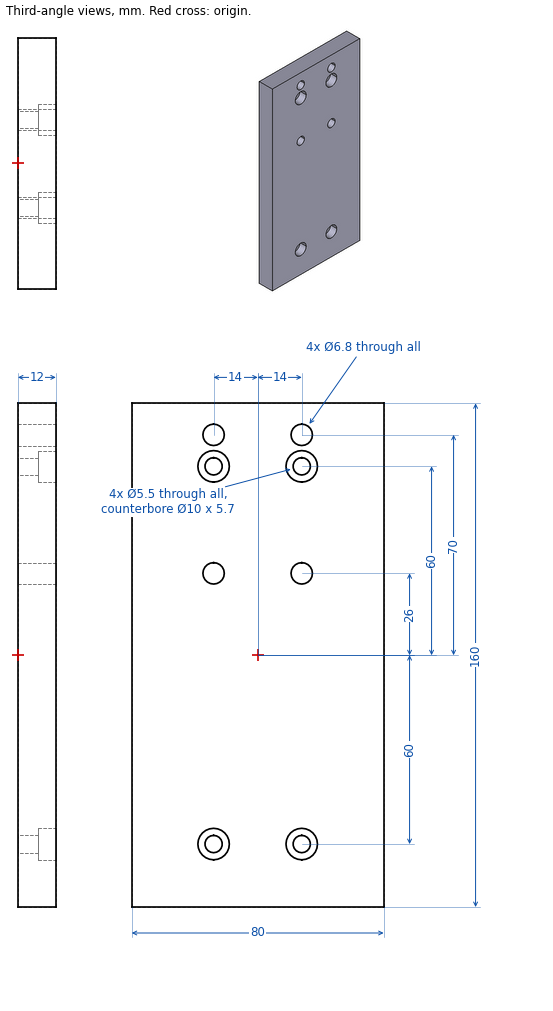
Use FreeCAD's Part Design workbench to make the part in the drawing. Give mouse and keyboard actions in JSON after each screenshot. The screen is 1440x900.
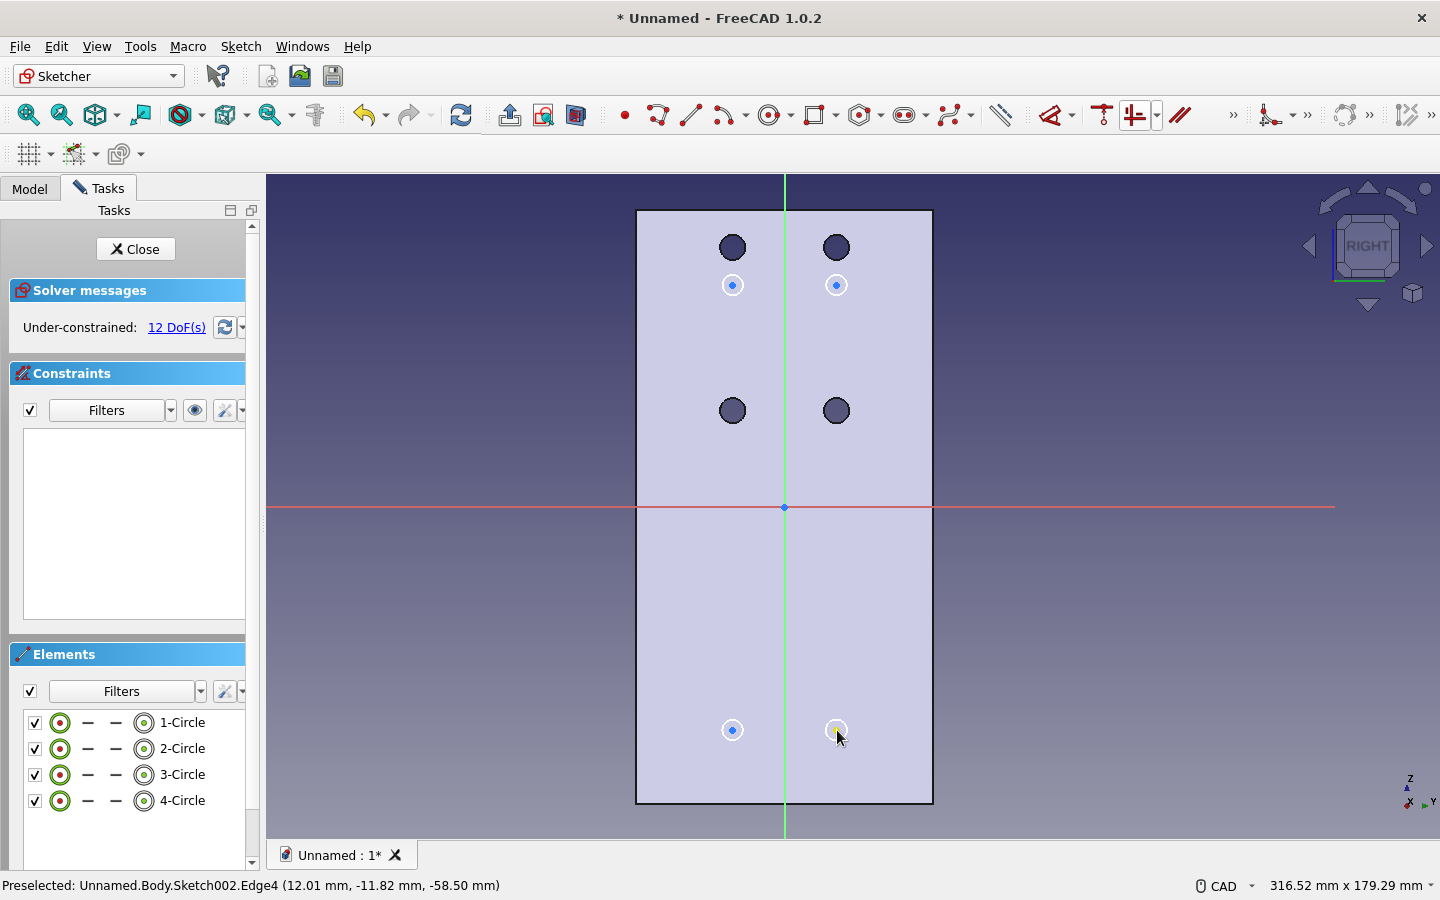
{"action": "scroll", "coordinate": [844, 278], "scroll_direction": "up", "scroll_amount": 2}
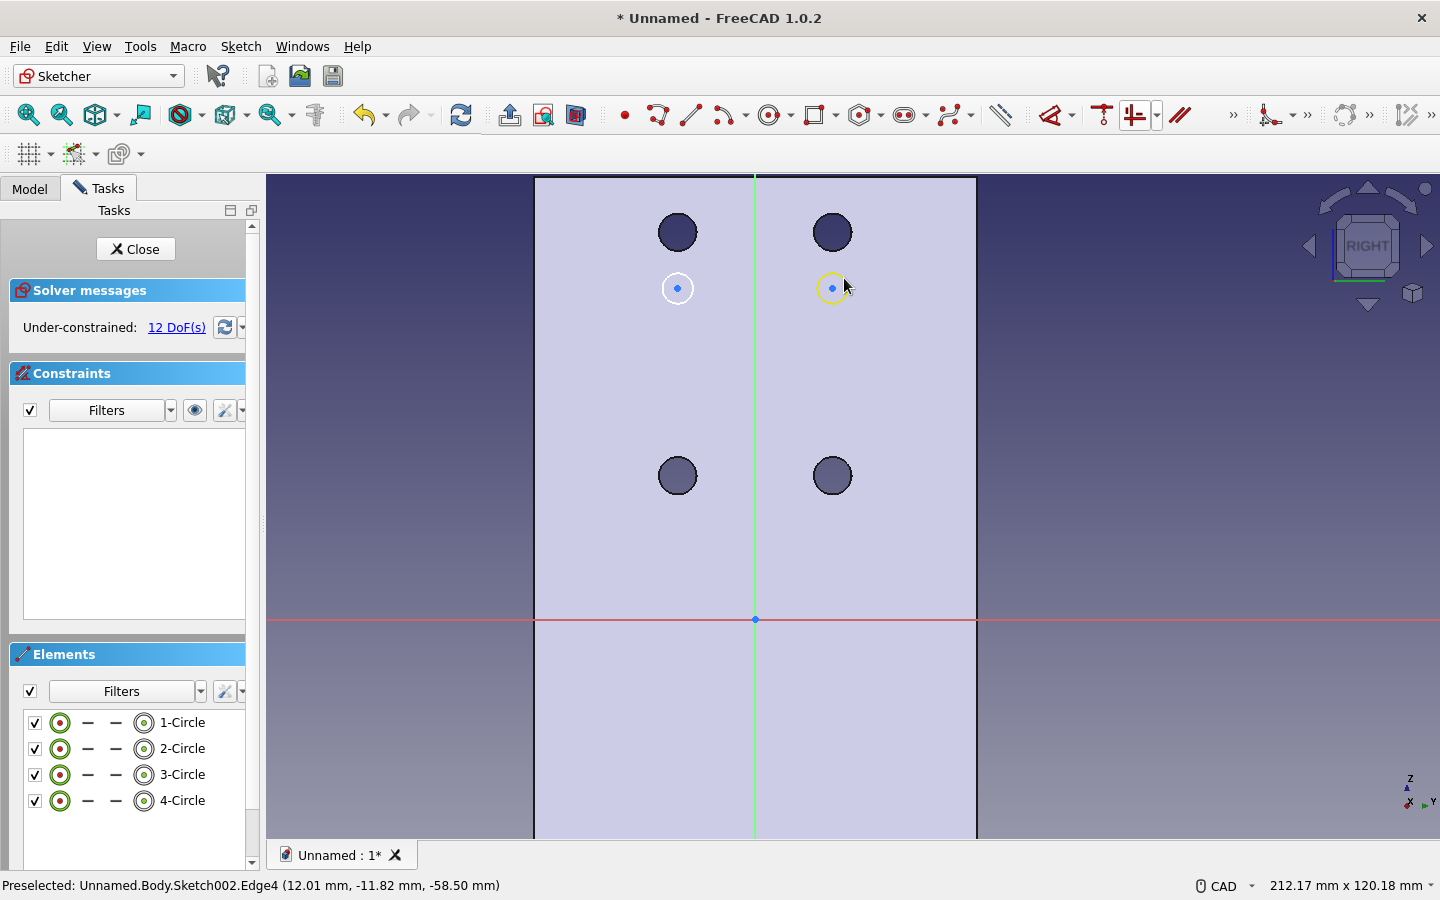
{"action": "left_click", "coordinate": [843, 278]}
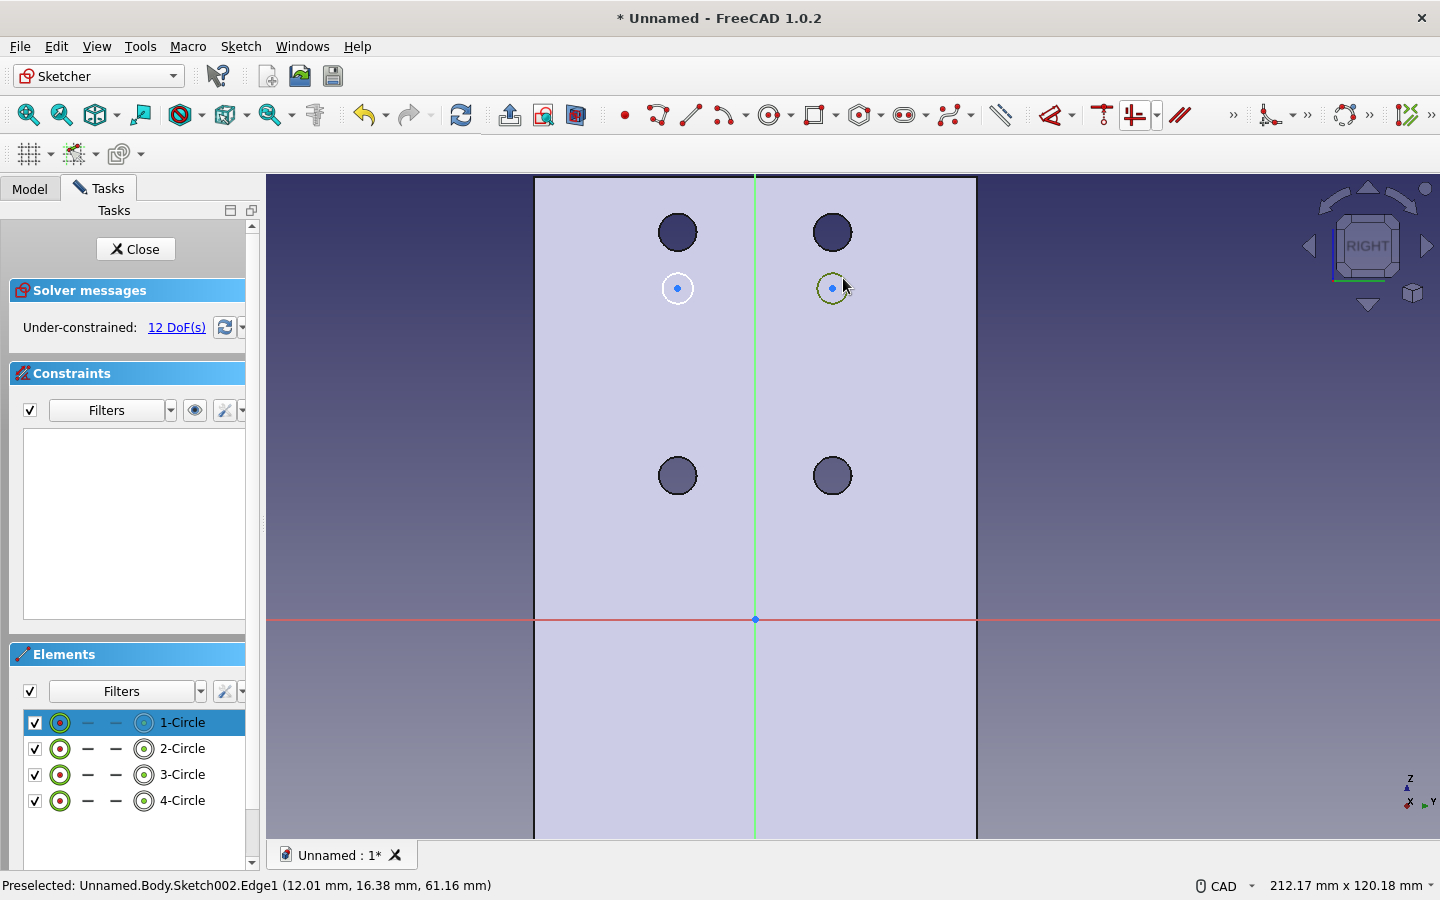
{"action": "left_click", "coordinate": [688, 278]}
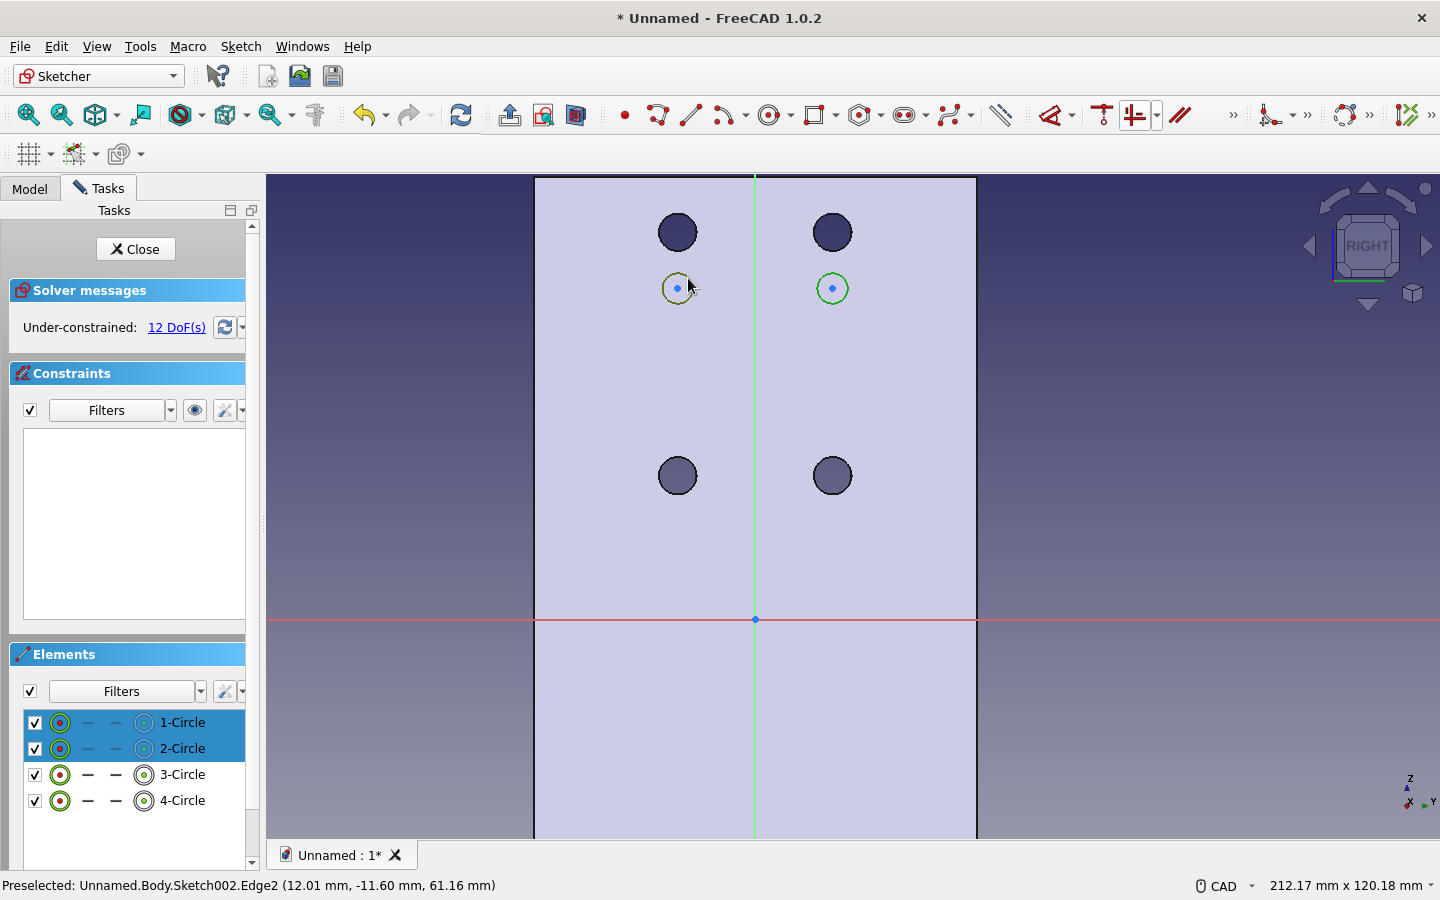
{"action": "scroll", "coordinate": [844, 276], "scroll_direction": "down", "scroll_amount": 2}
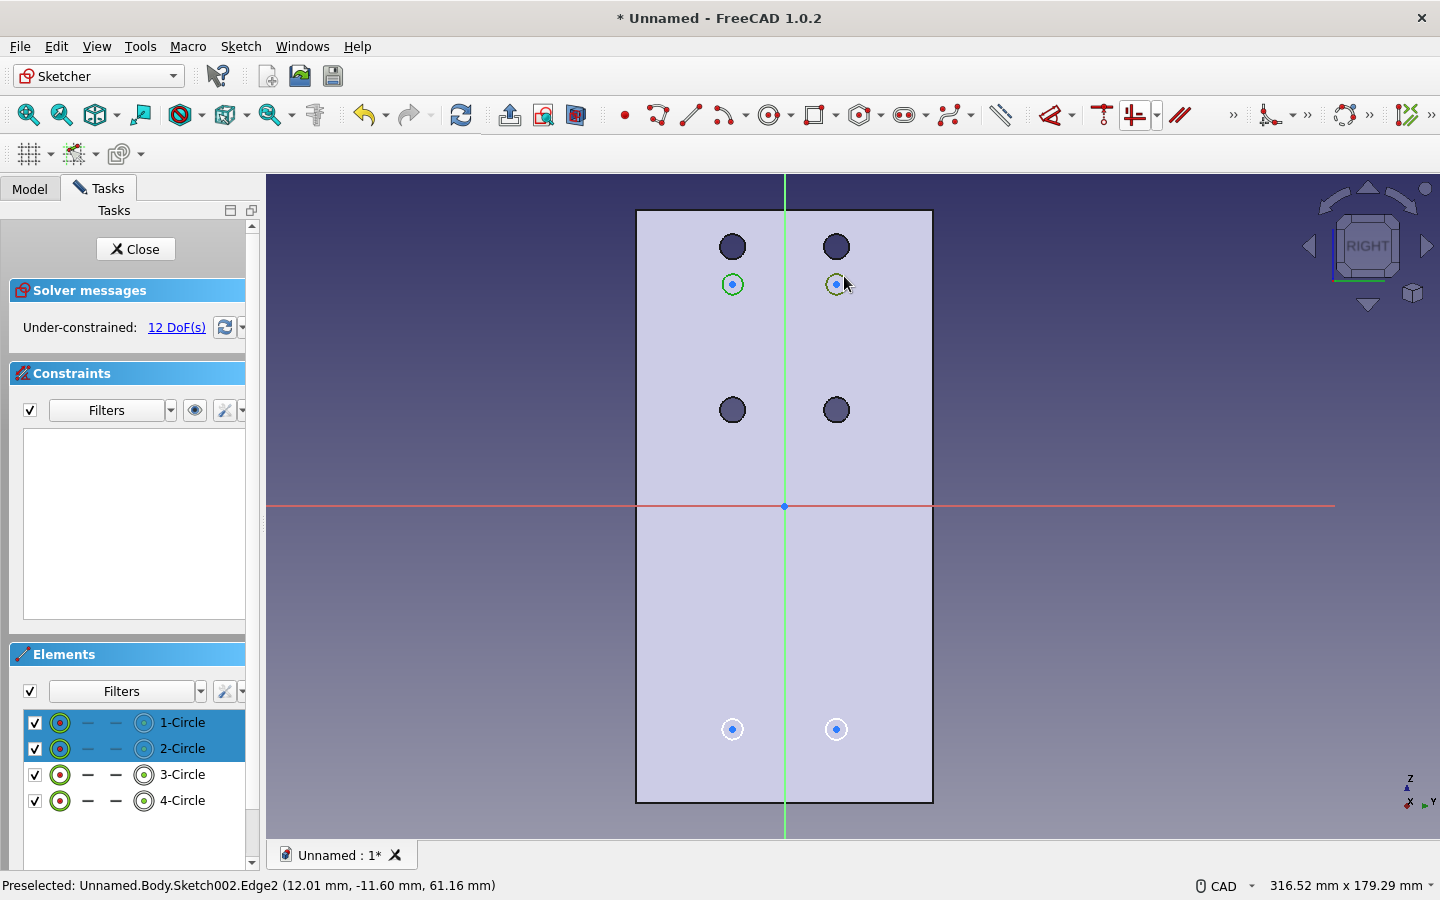
{"action": "scroll", "coordinate": [844, 722], "scroll_direction": "up", "scroll_amount": 2}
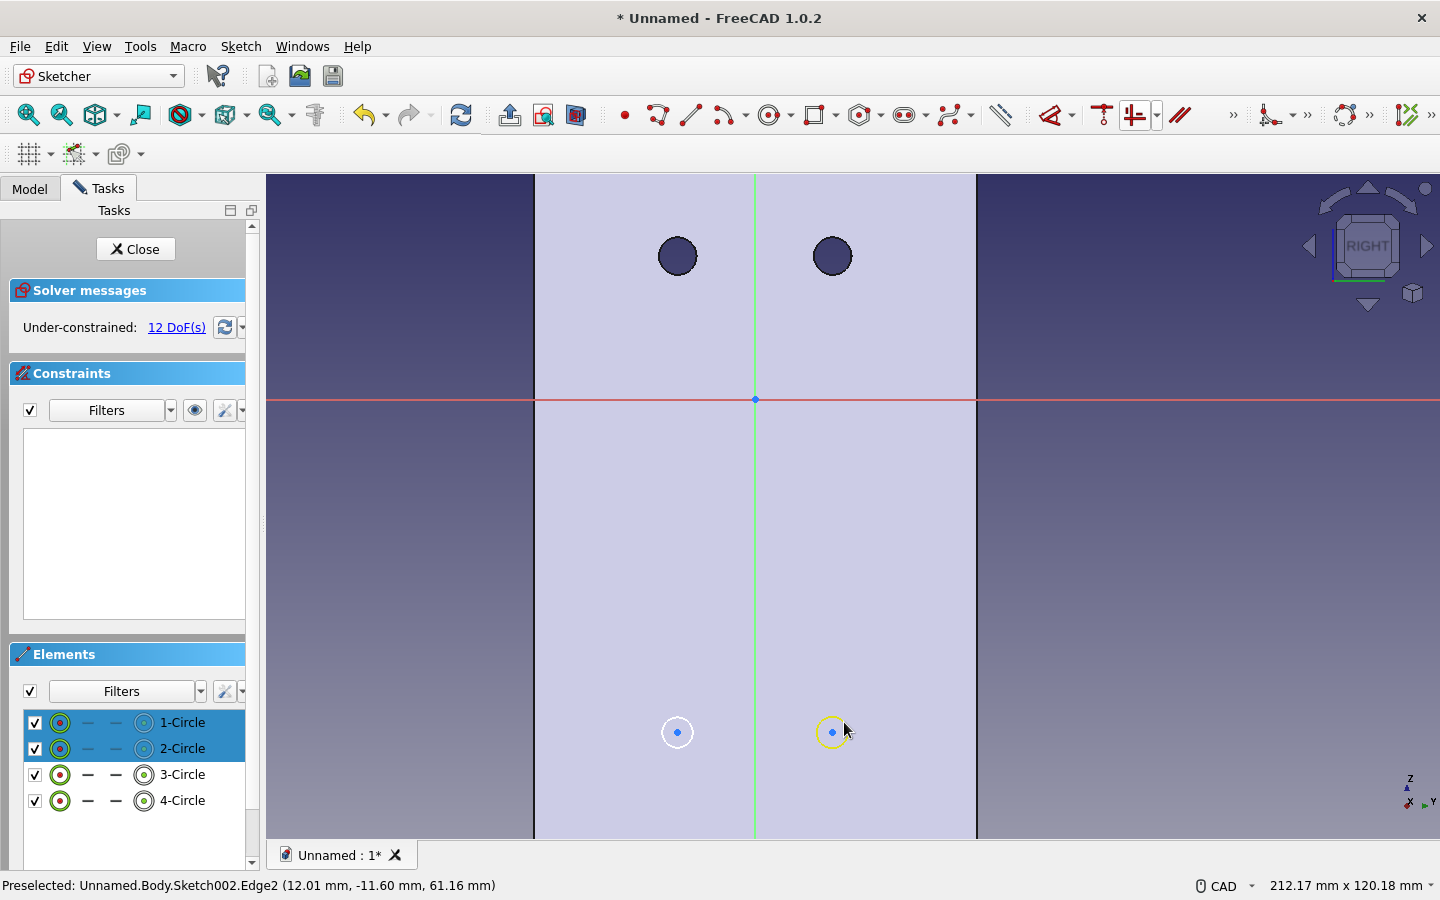
{"action": "left_click", "coordinate": [843, 721]}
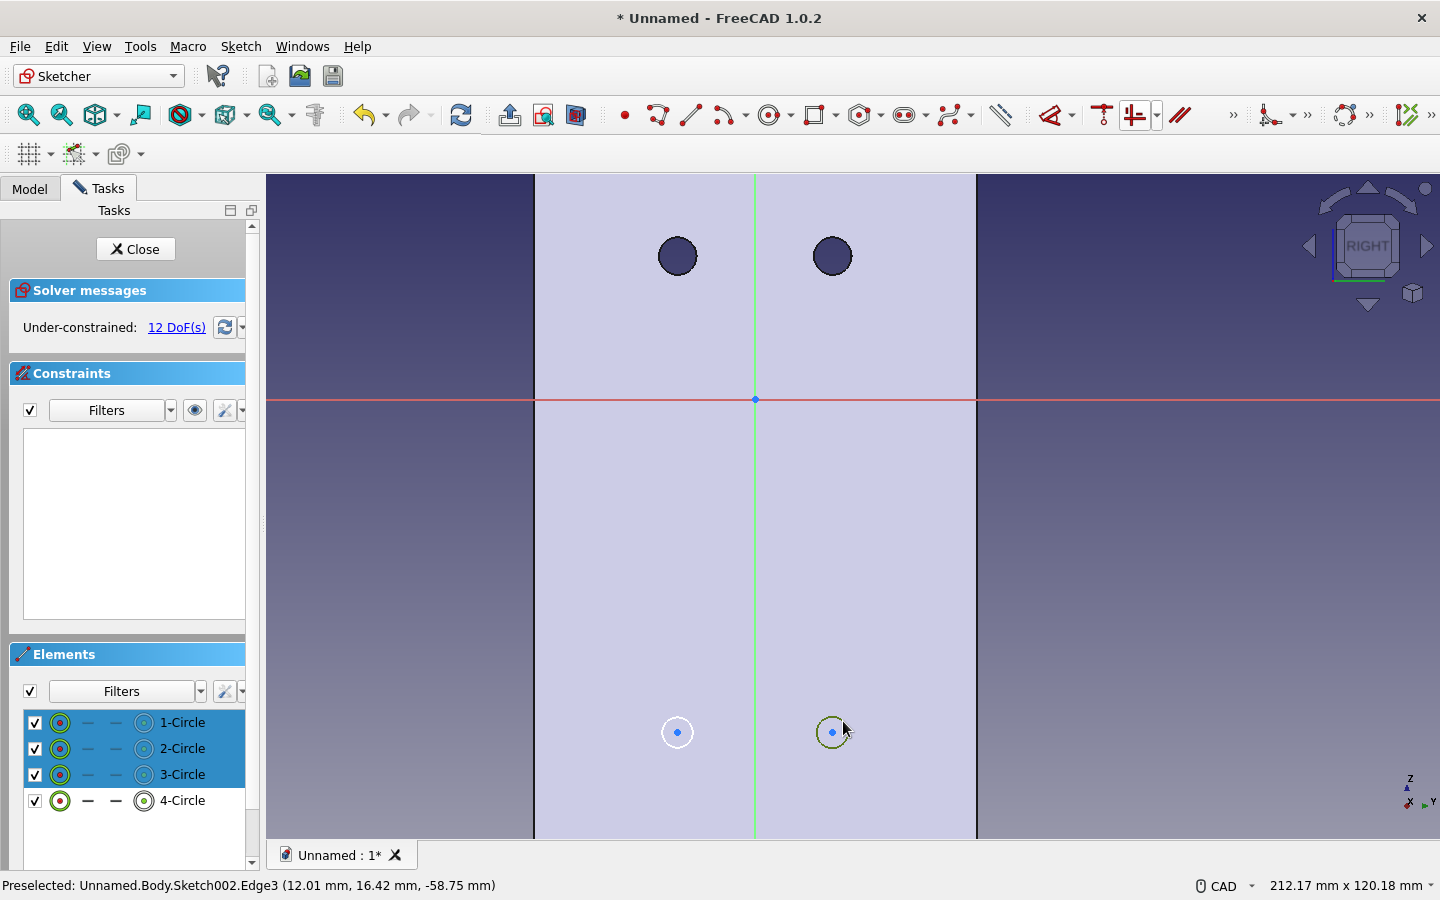
{"action": "left_click", "coordinate": [688, 722]}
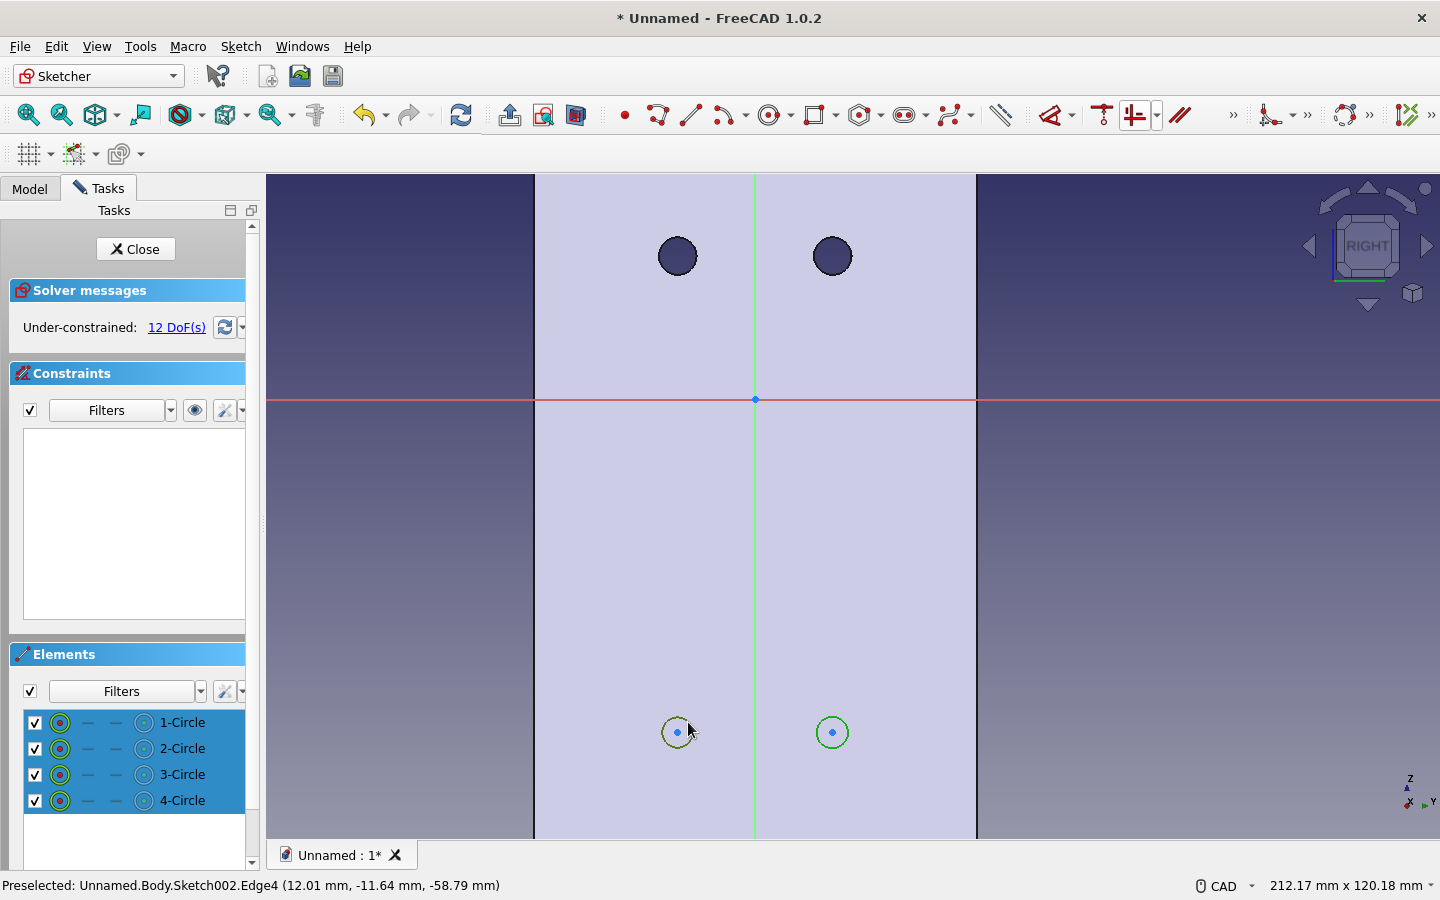
{"action": "key", "text": "e"}